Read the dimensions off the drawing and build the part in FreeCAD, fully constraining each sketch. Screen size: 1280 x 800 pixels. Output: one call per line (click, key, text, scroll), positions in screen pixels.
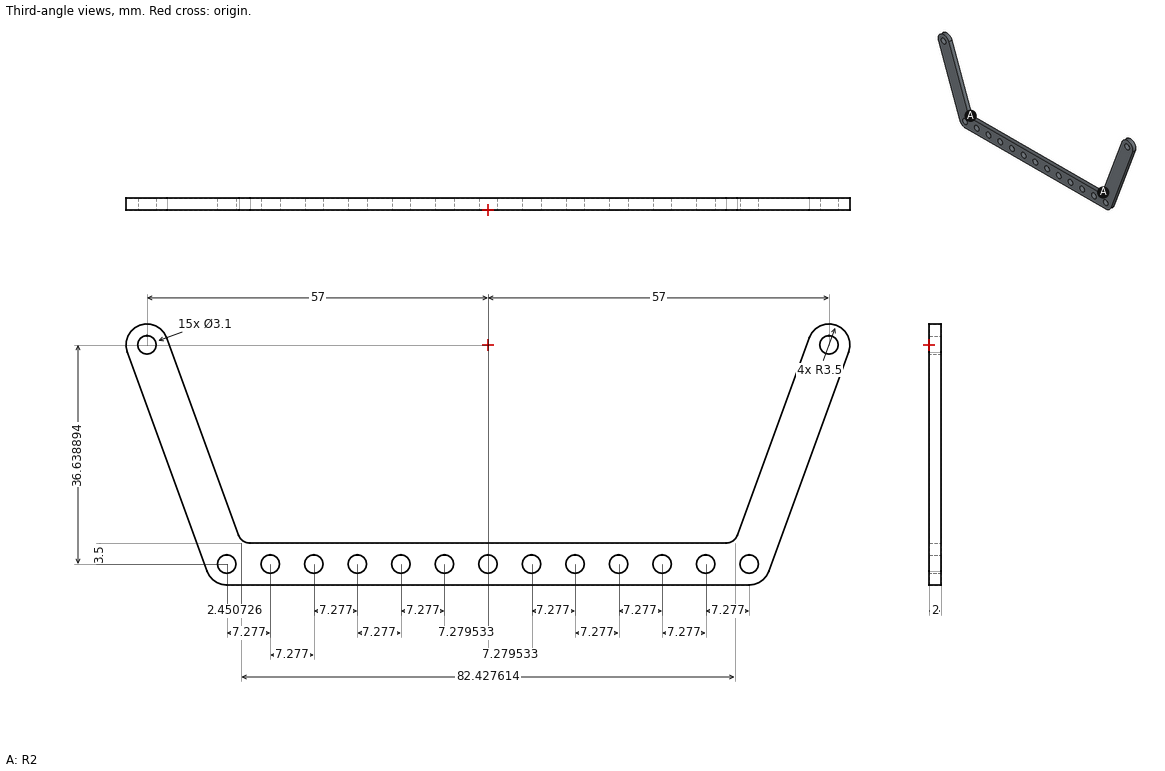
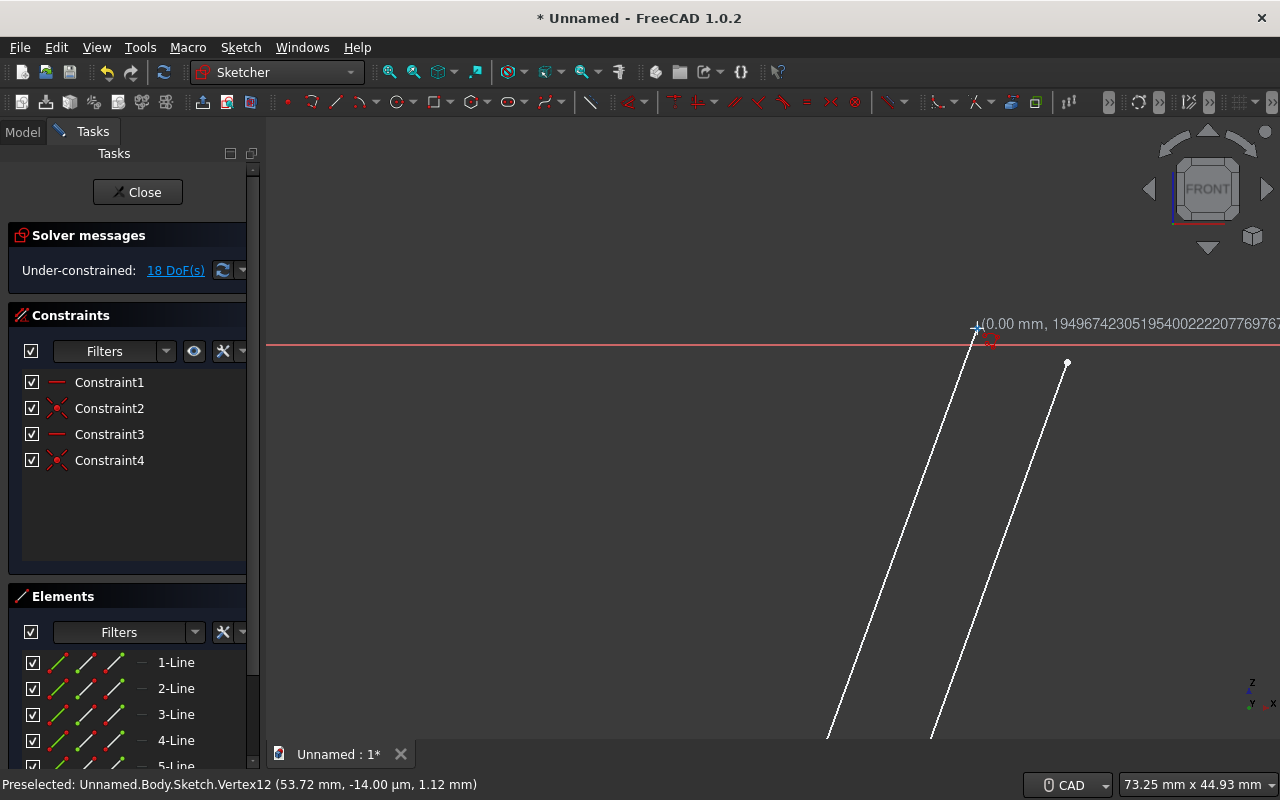
key(g)
key(3)
key(a)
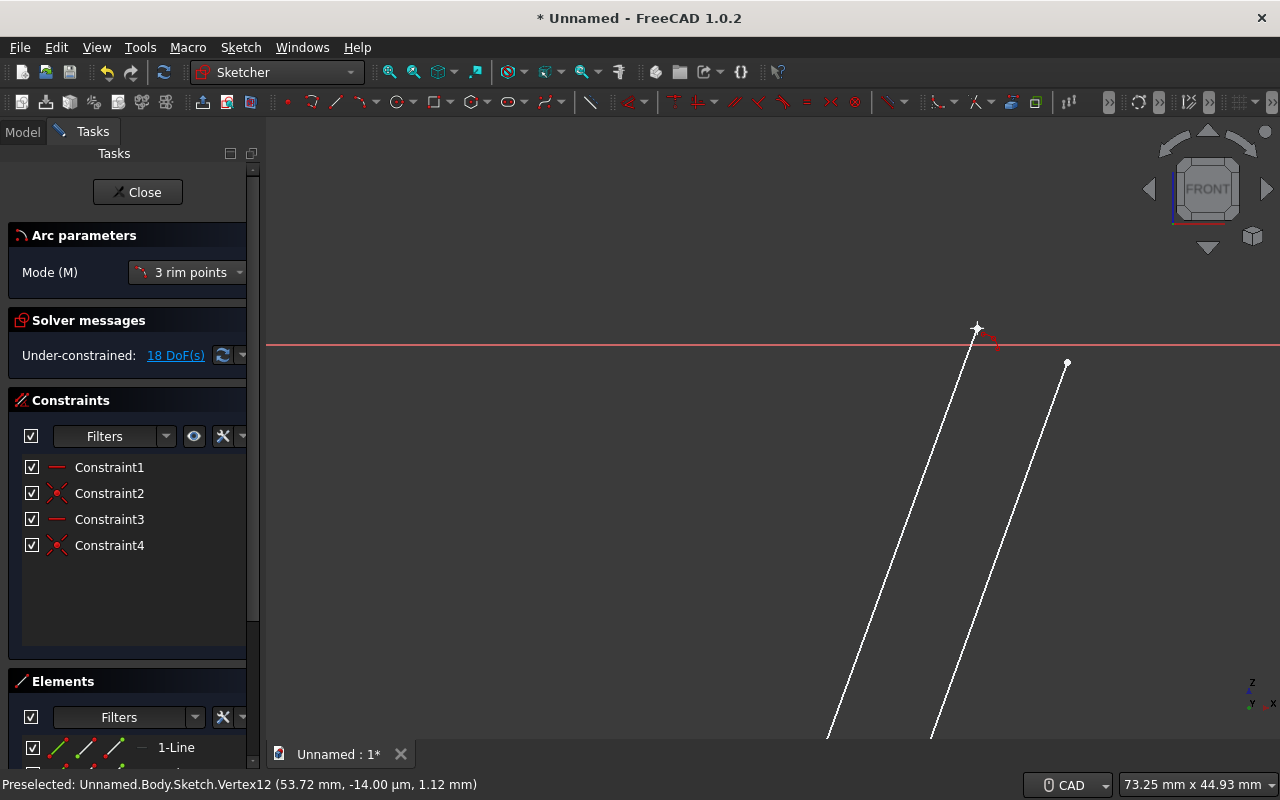
scroll(979, 328, down, 5)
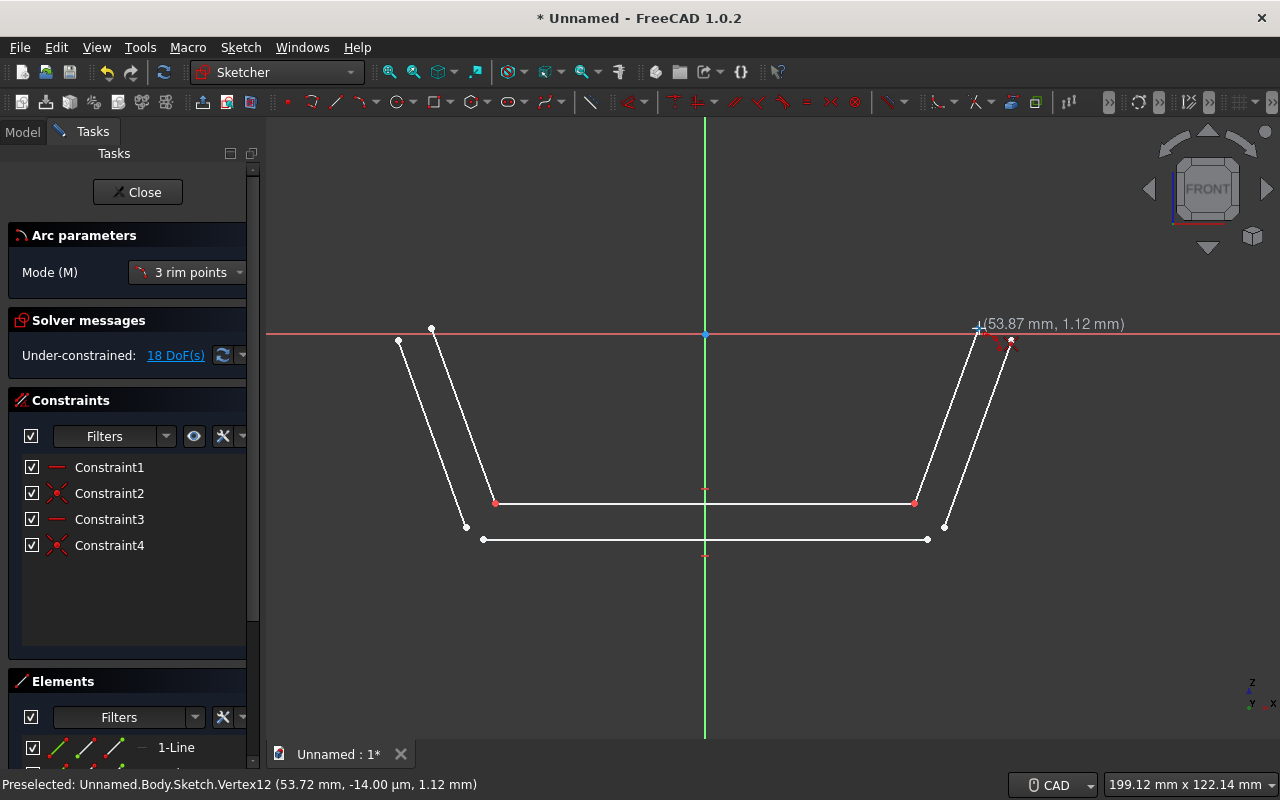
click(944, 528)
click(927, 540)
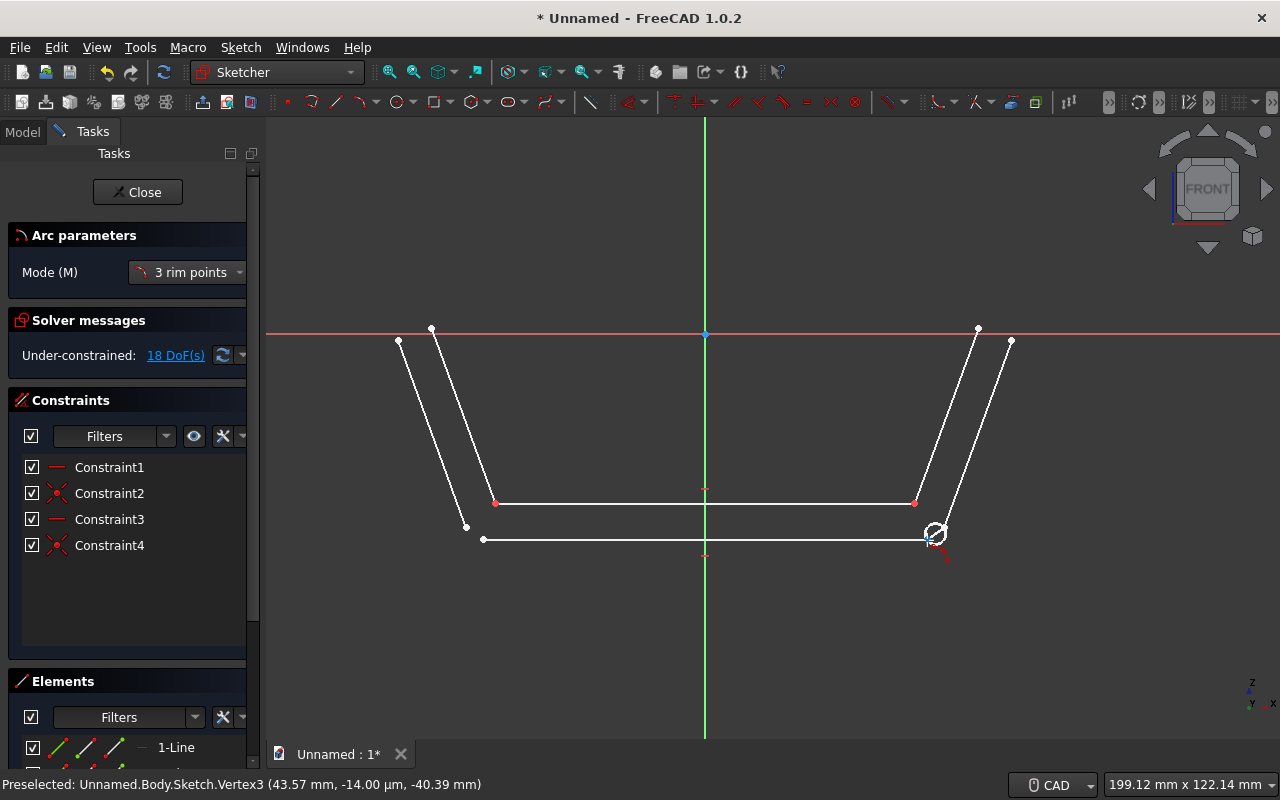
scroll(938, 535, up, 8)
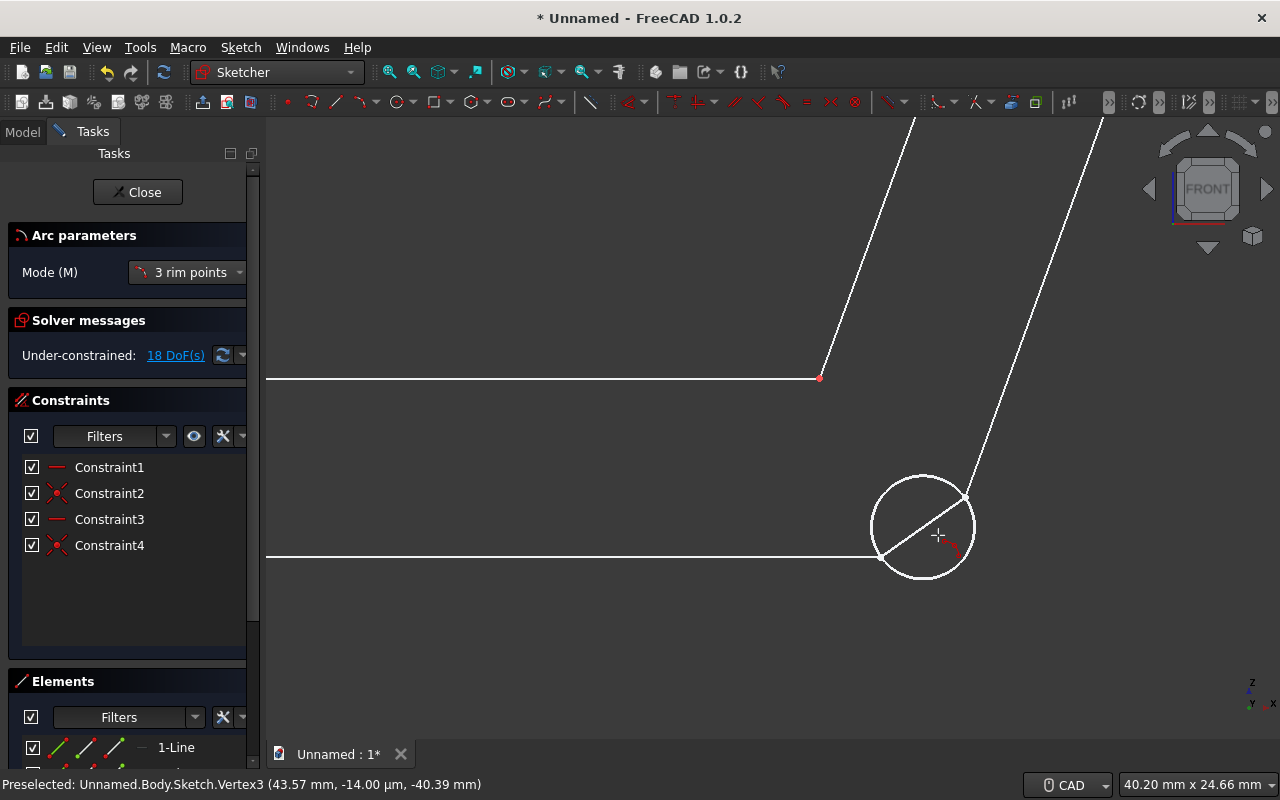
click(934, 535)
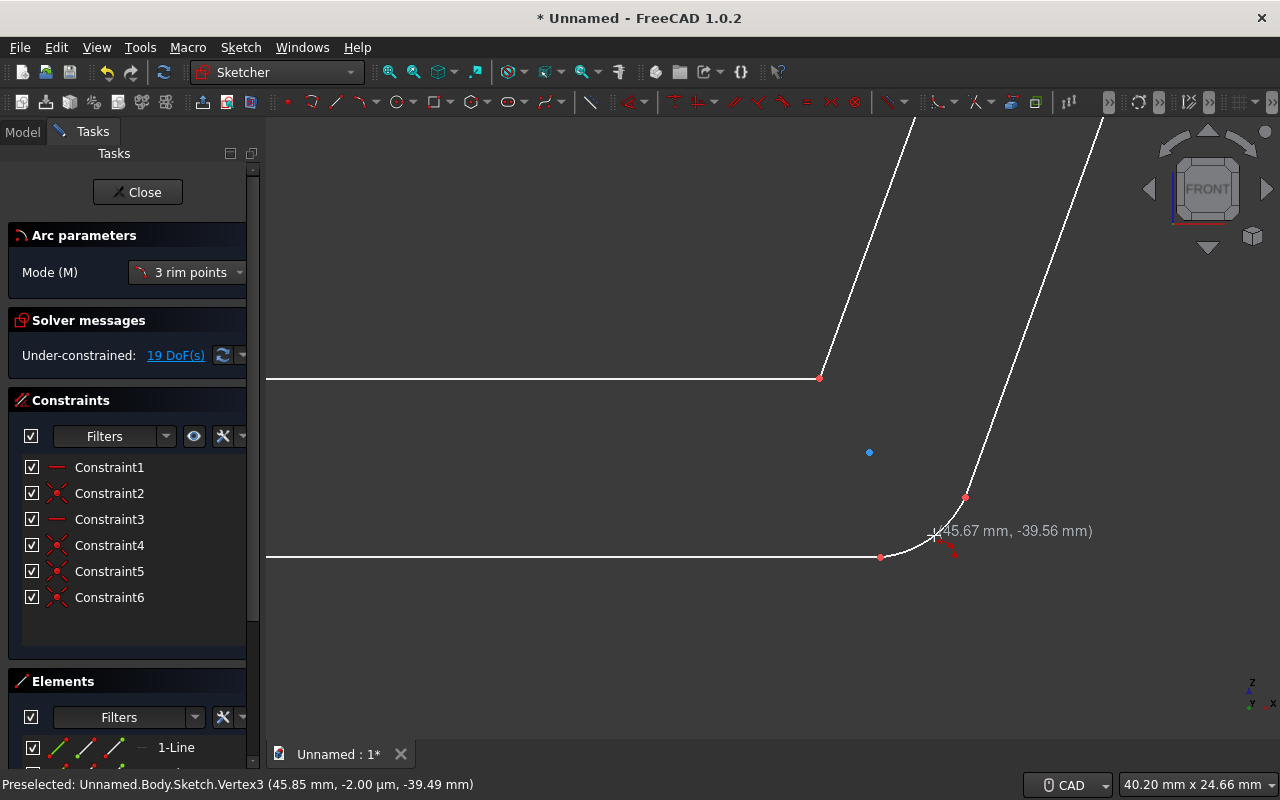
scroll(938, 536, down, 8)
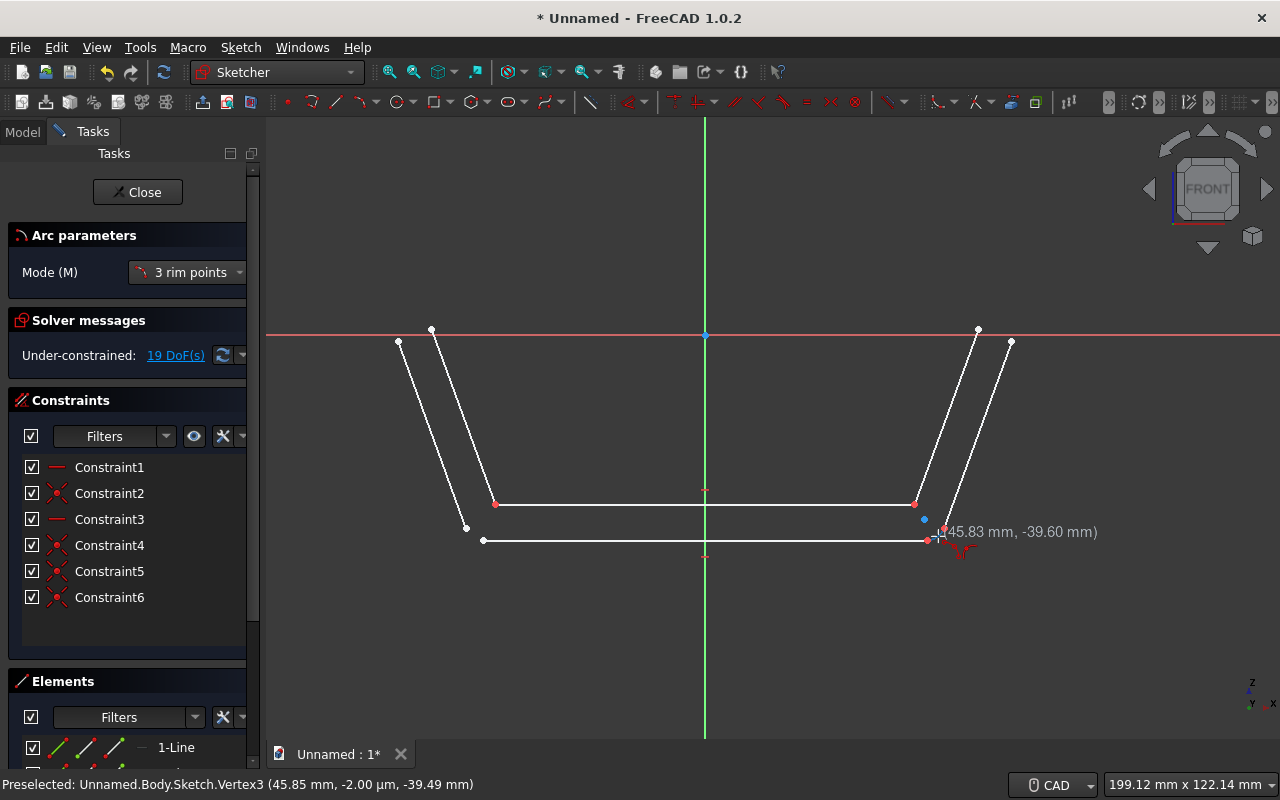
click(483, 541)
click(466, 529)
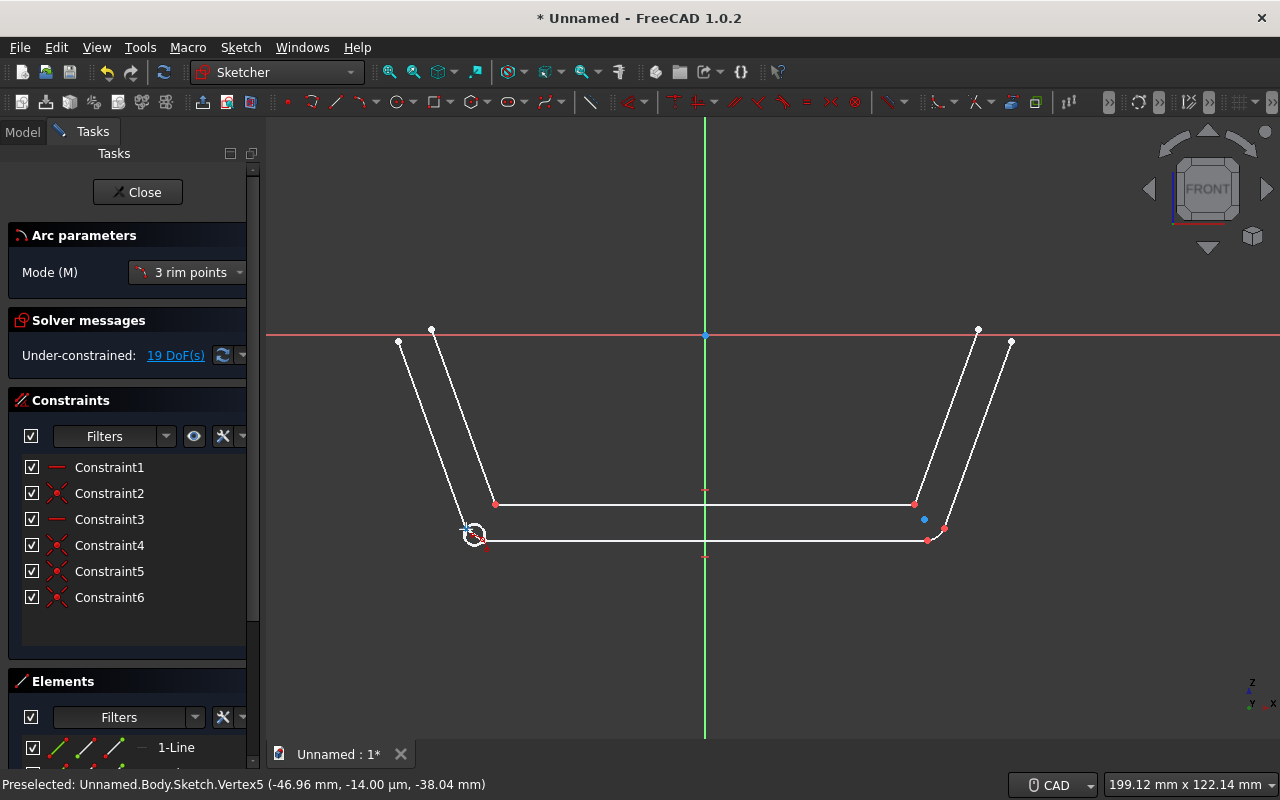
scroll(473, 536, up, 8)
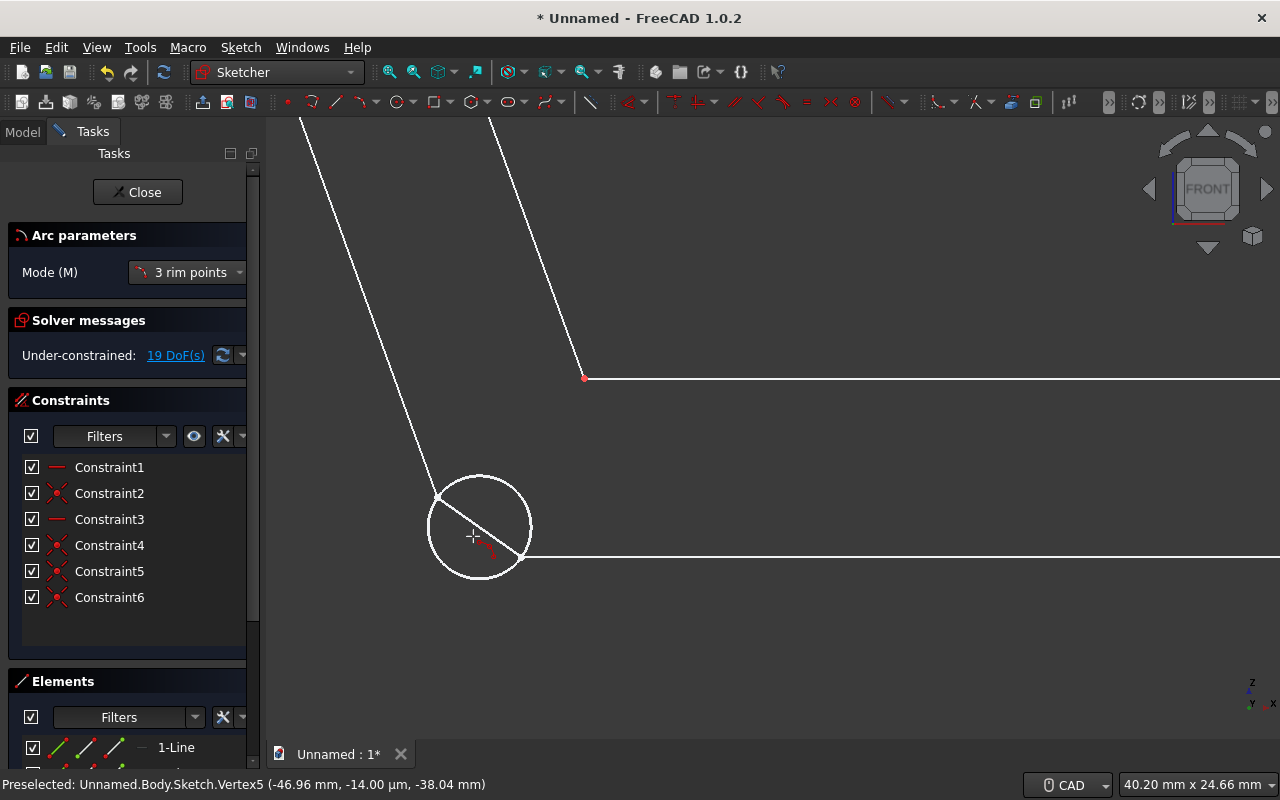
click(470, 535)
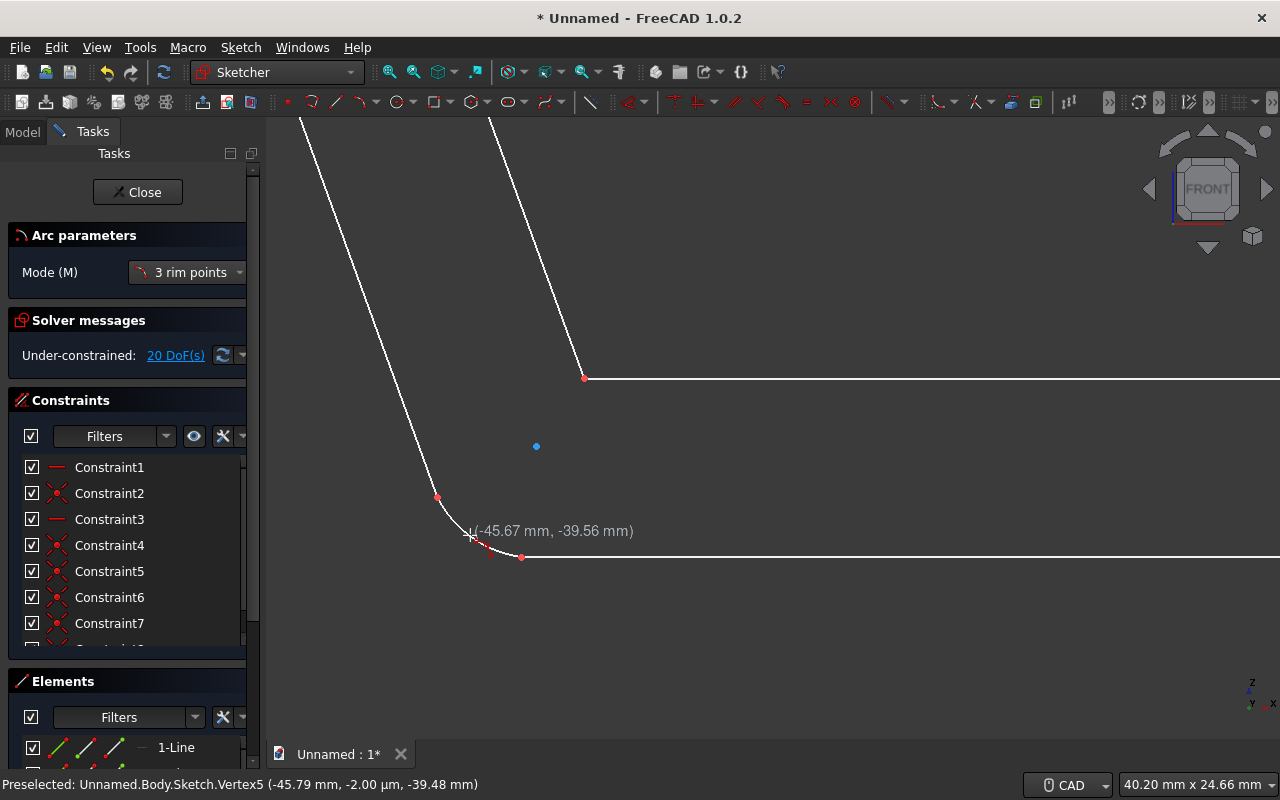
scroll(472, 536, down, 8)